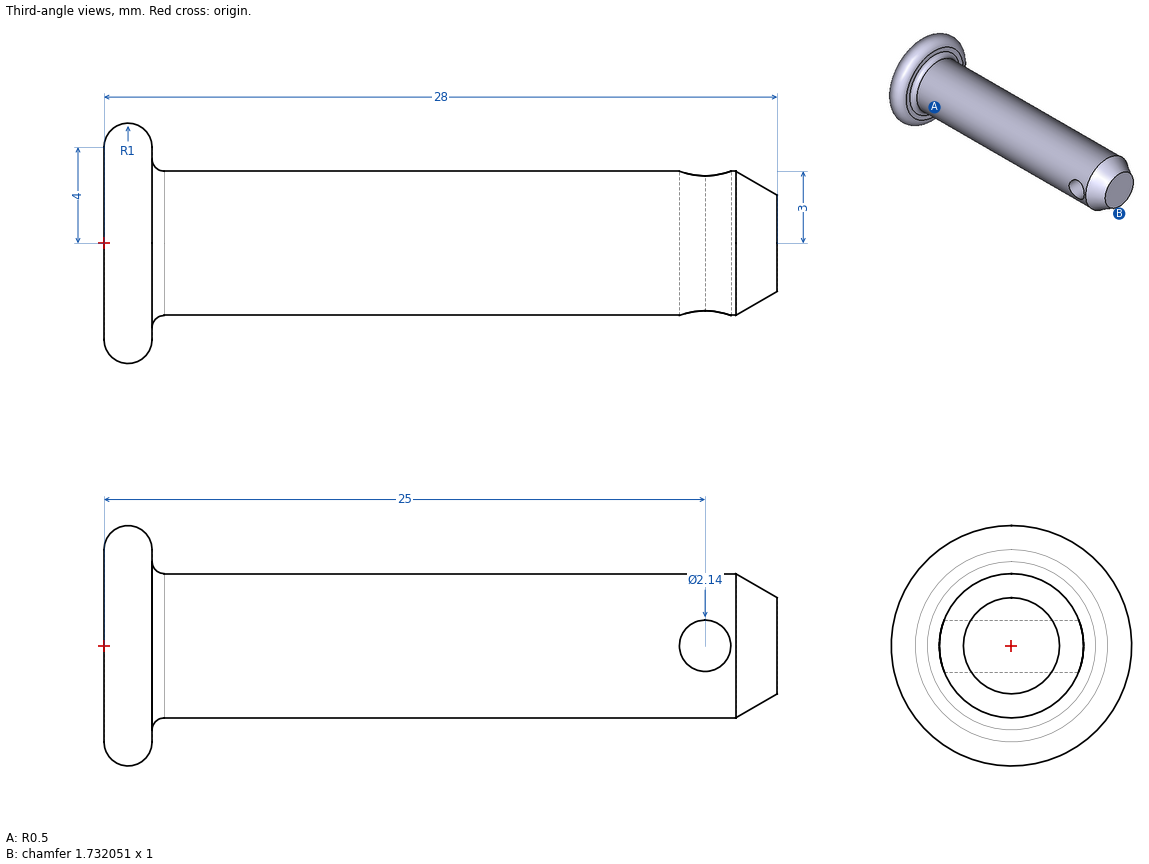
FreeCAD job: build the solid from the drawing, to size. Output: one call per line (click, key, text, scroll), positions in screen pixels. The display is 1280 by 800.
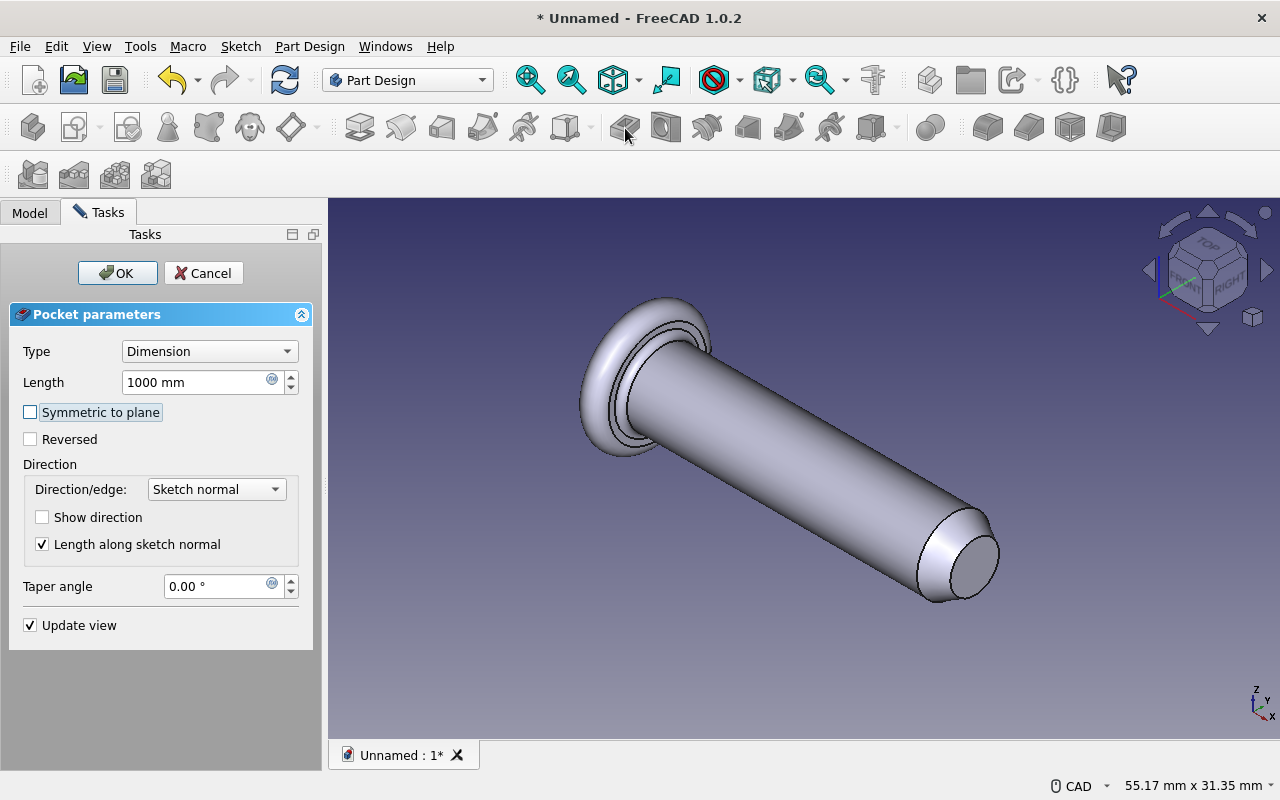
click(31, 412)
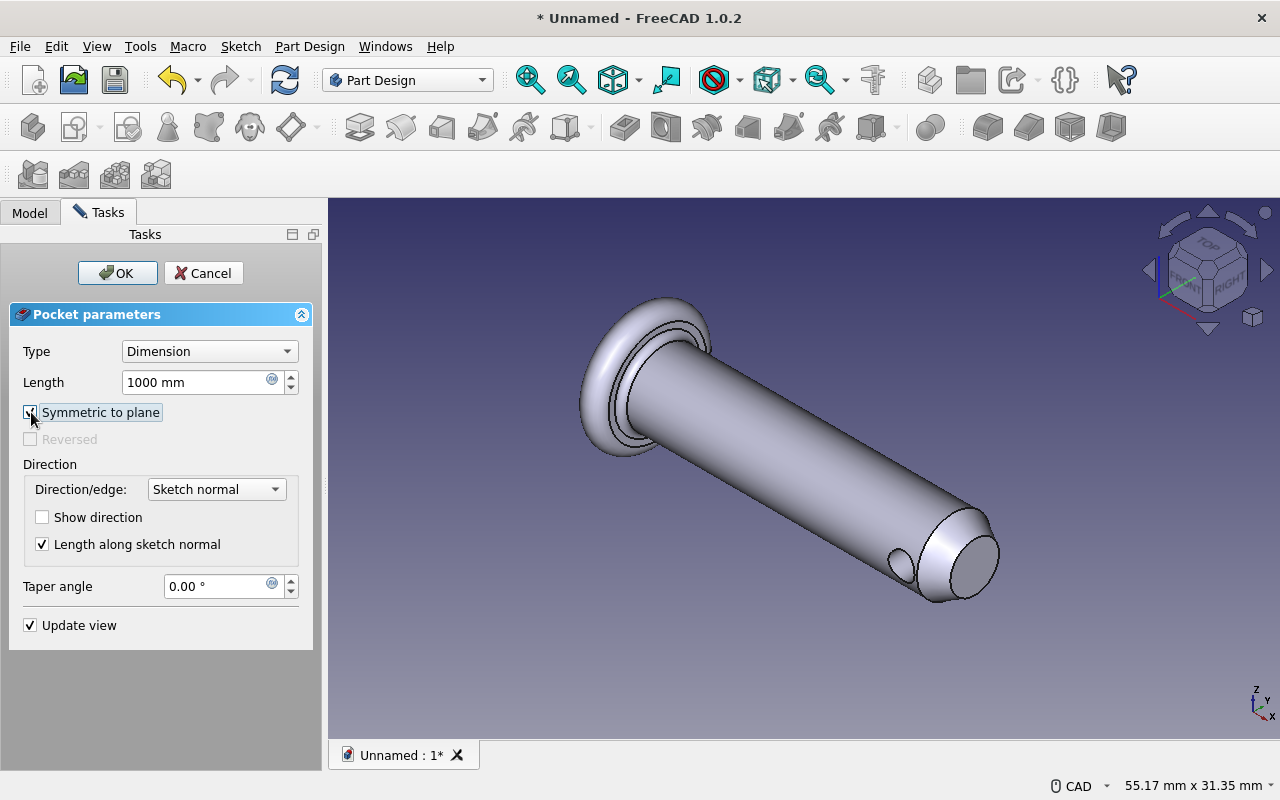
click(118, 273)